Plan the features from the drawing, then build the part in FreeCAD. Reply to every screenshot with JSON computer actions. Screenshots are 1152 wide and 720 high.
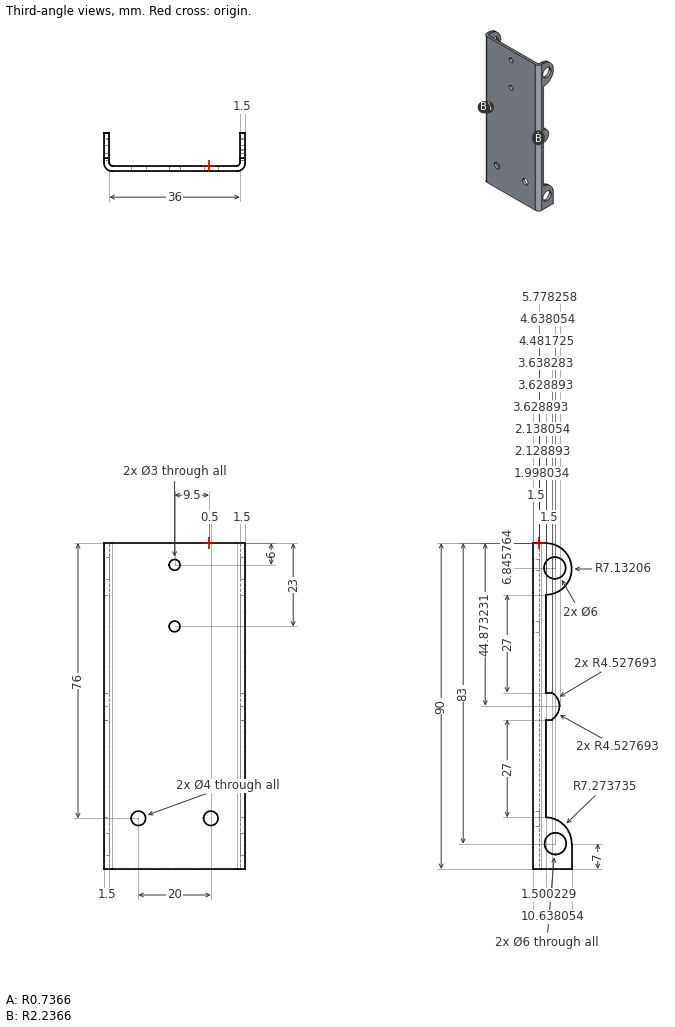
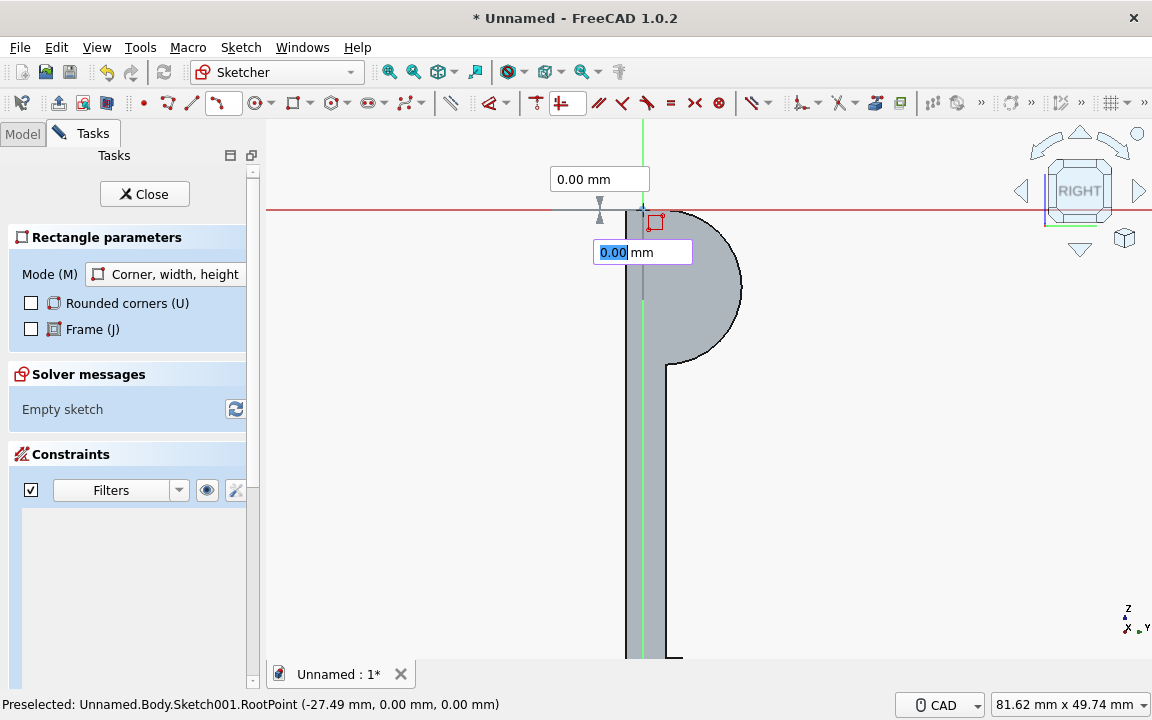
{"action": "scroll", "coordinate": [644, 209], "scroll_direction": "down", "scroll_amount": 5}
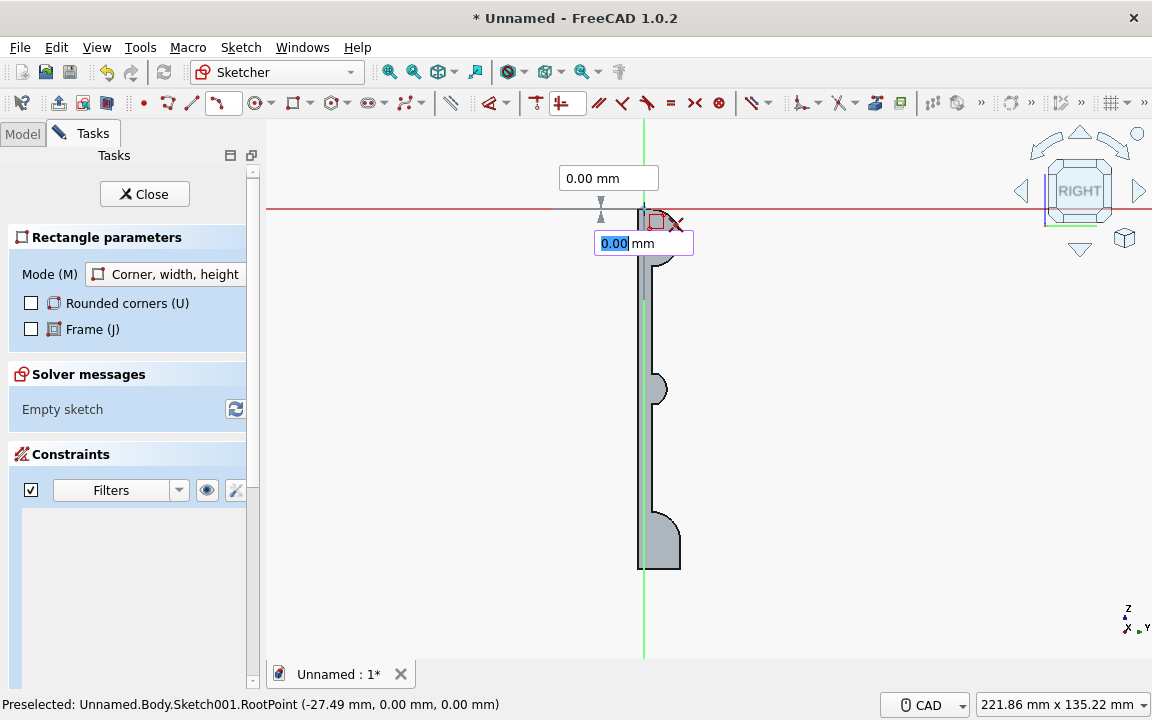
{"action": "scroll", "coordinate": [638, 569], "scroll_direction": "up", "scroll_amount": 5}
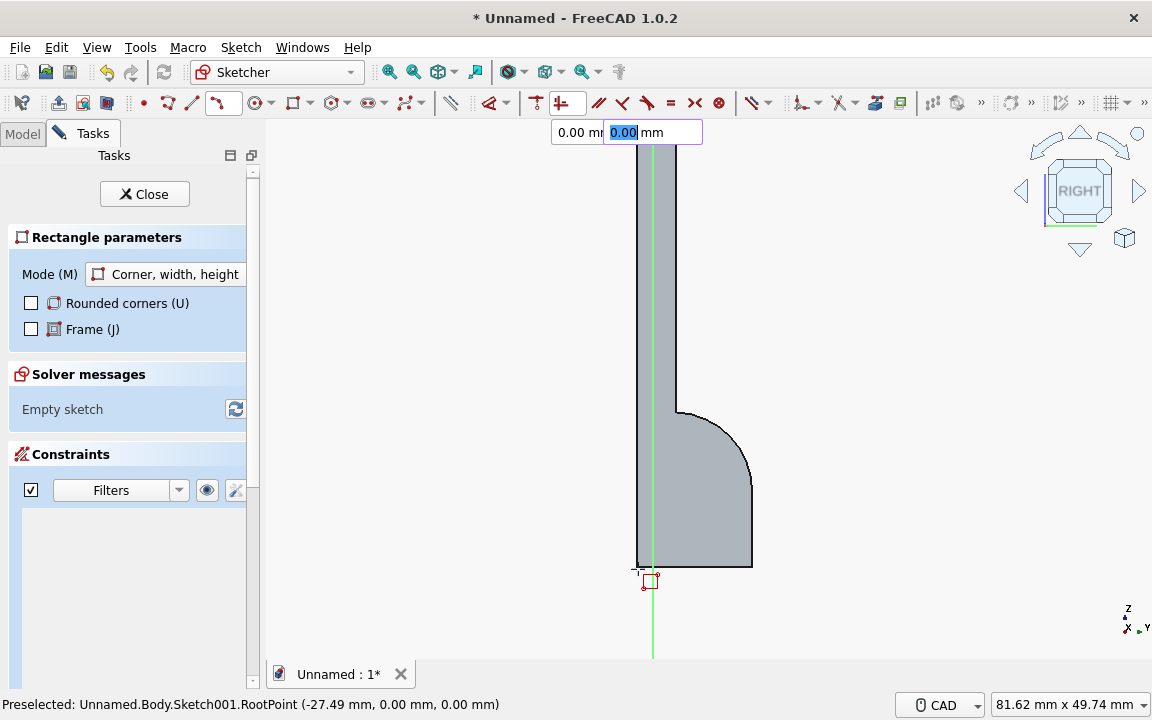
{"action": "left_click", "coordinate": [637, 567]}
{"action": "key", "text": "Escape"}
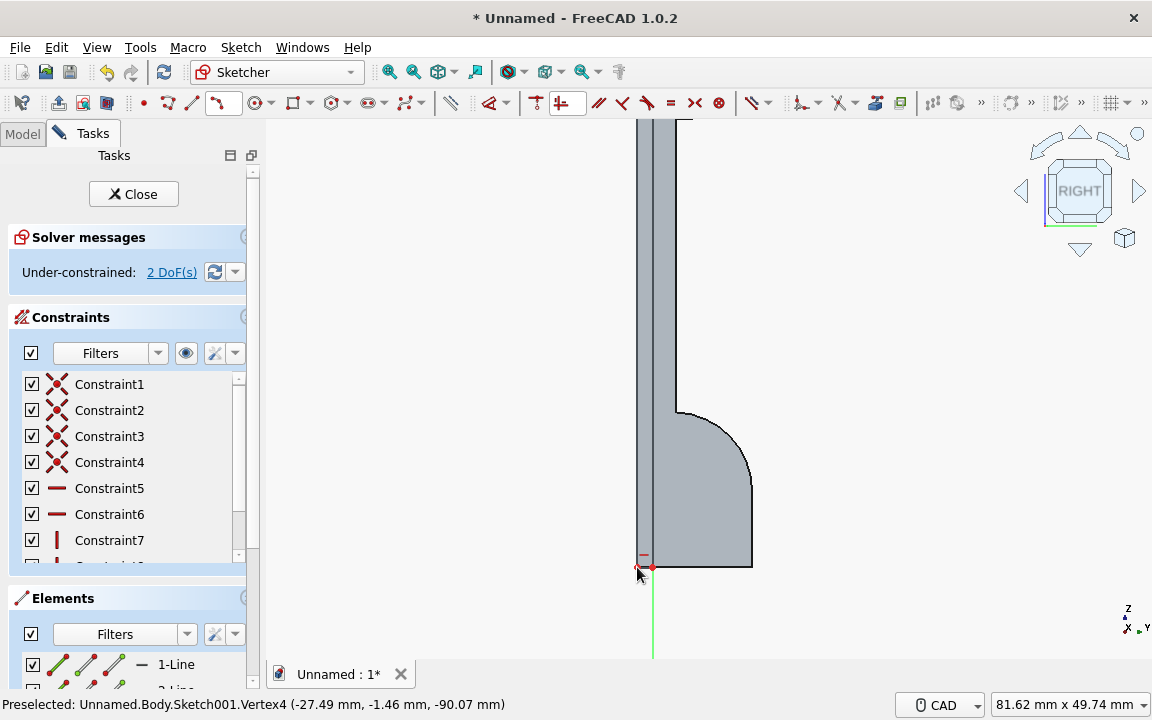
{"action": "key", "text": "d"}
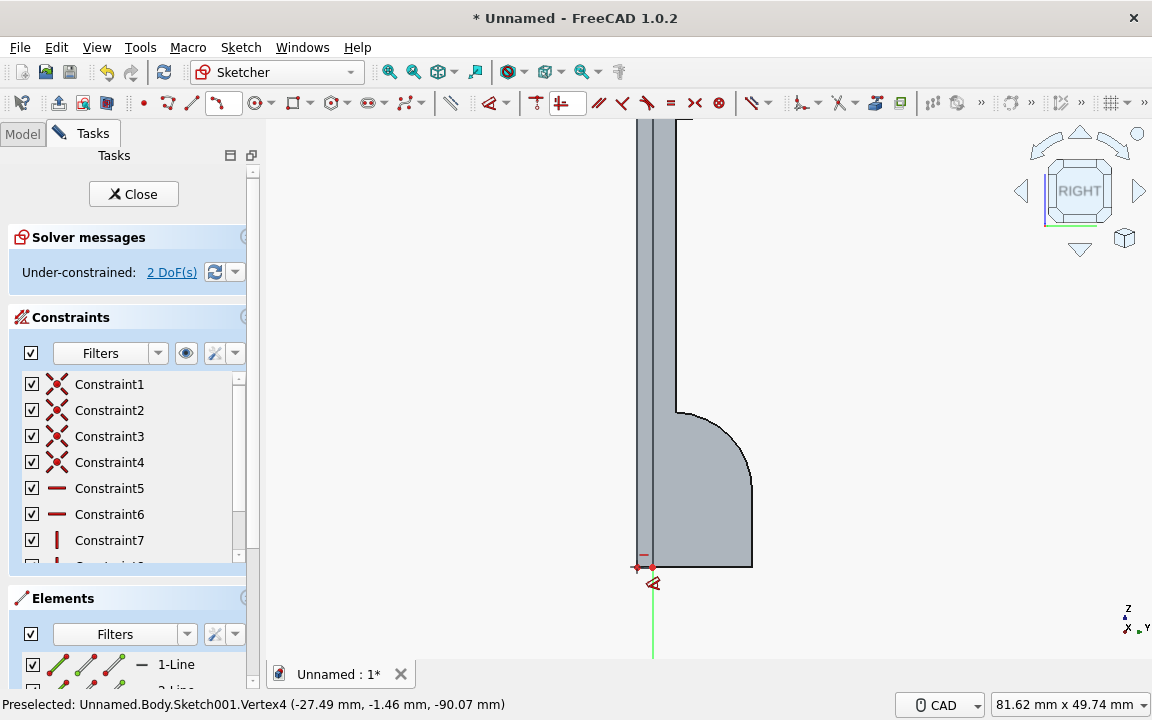
{"action": "left_click", "coordinate": [637, 275]}
{"action": "left_click", "coordinate": [603, 357]}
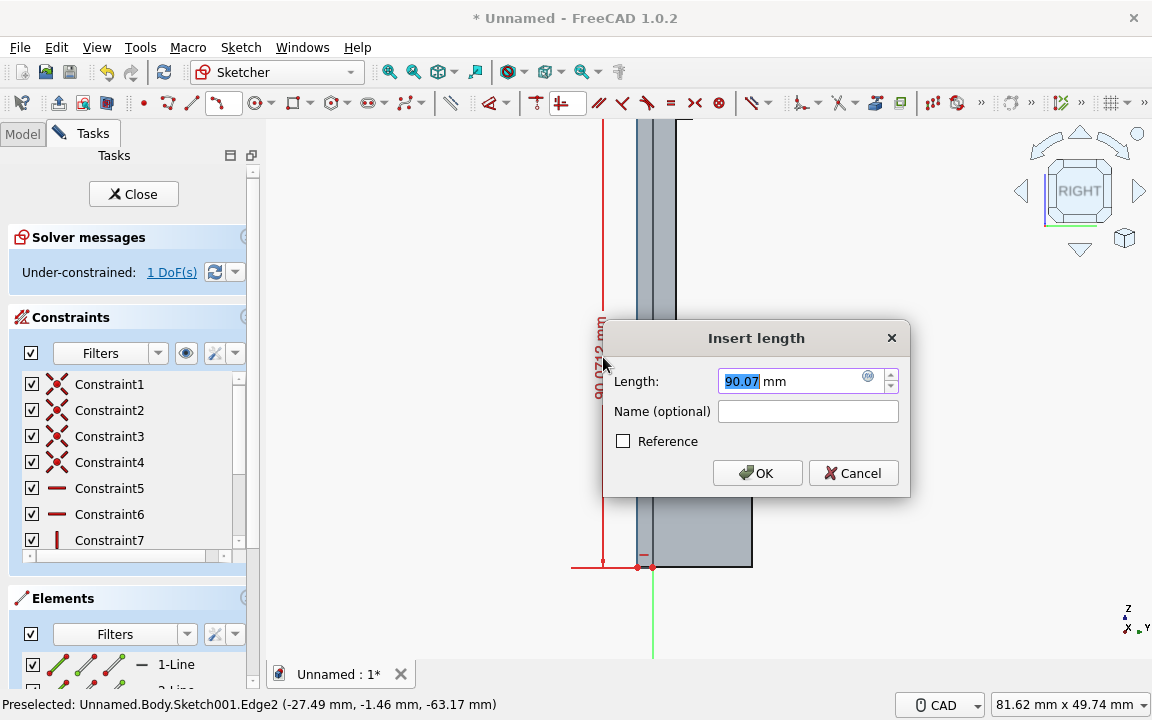
{"action": "type", "text": "90"}
{"action": "key", "text": "Return"}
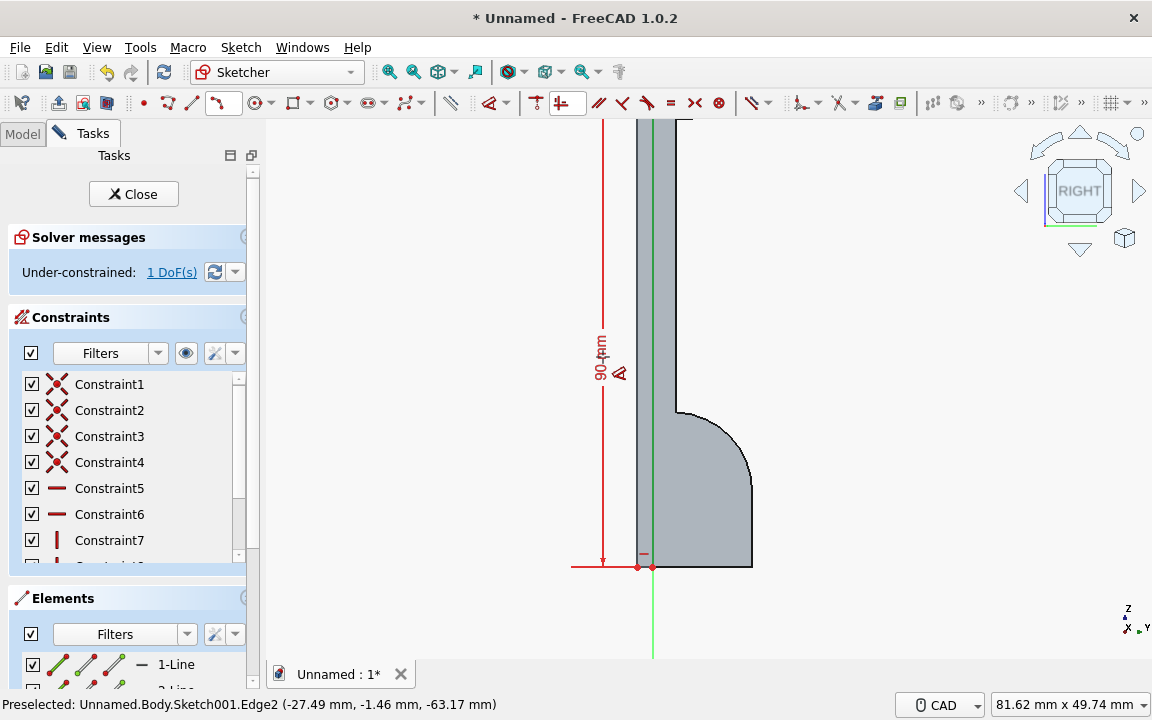
{"action": "scroll", "coordinate": [638, 570], "scroll_direction": "down", "scroll_amount": 5}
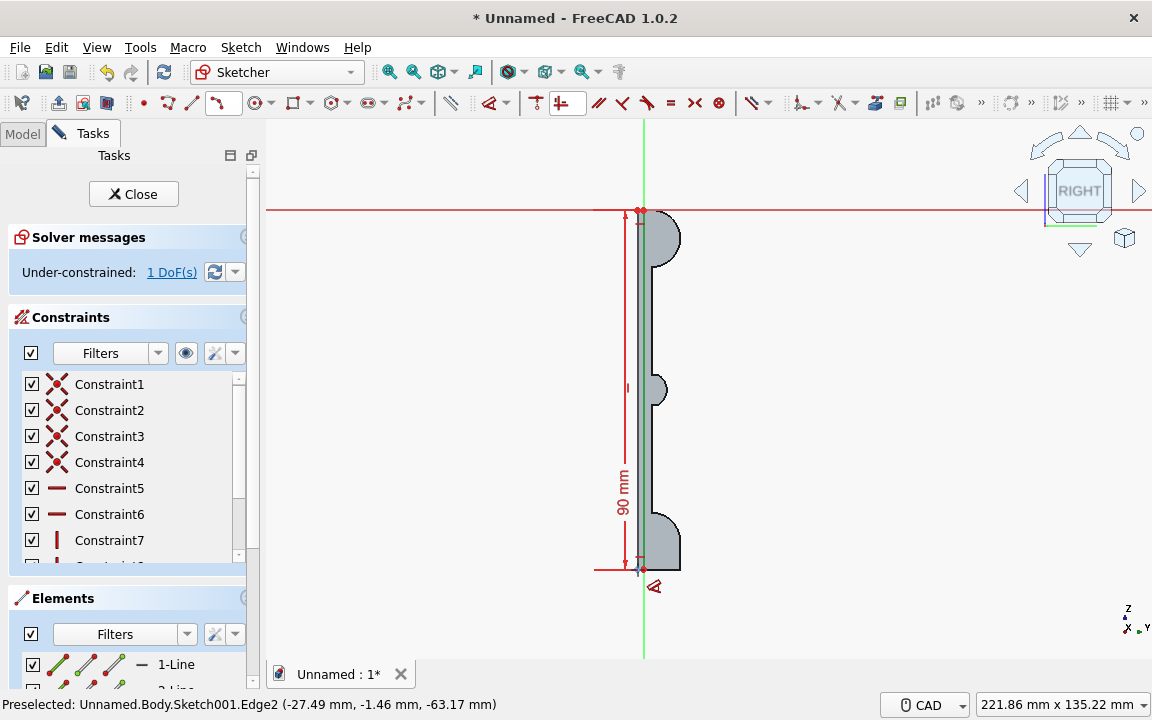
{"action": "scroll", "coordinate": [641, 210], "scroll_direction": "up", "scroll_amount": 10}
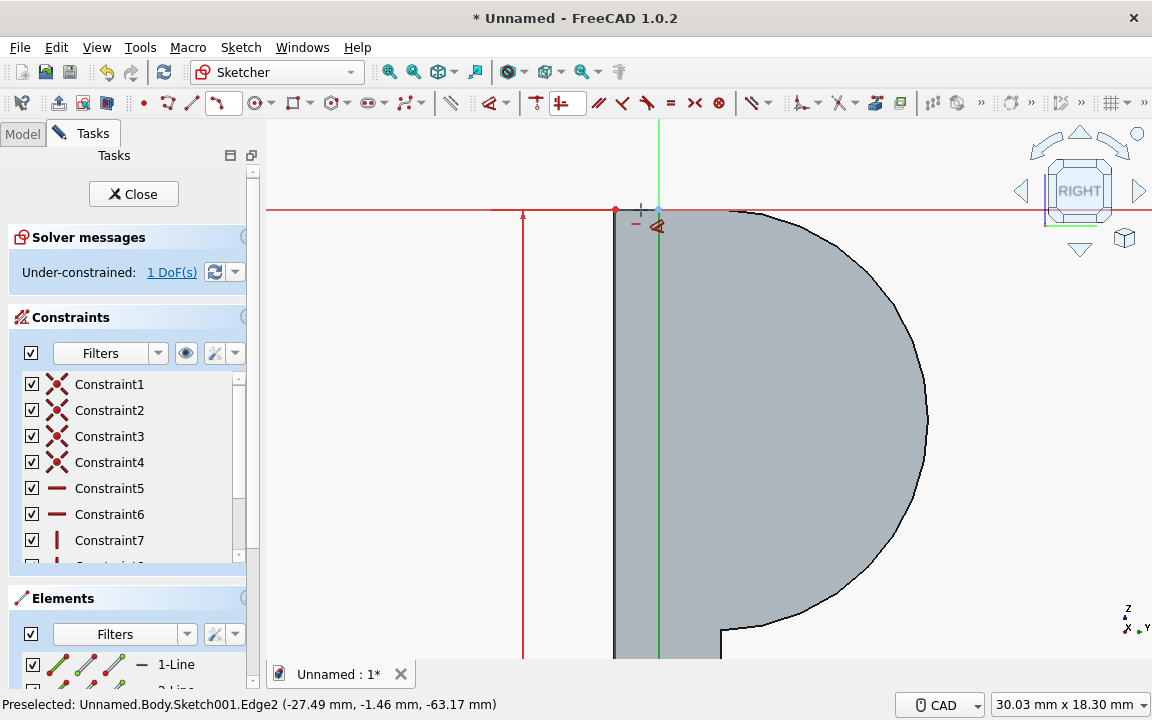
{"action": "left_click", "coordinate": [637, 210]}
{"action": "left_click", "coordinate": [637, 176]}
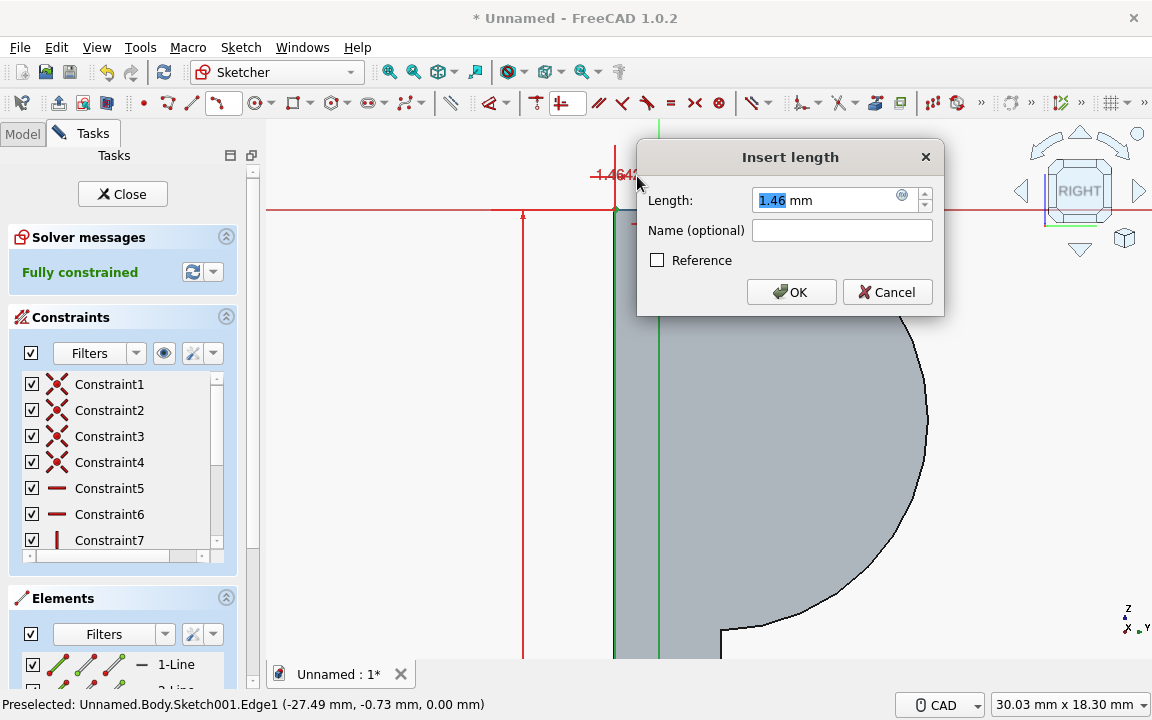
{"action": "type", "text": "1.5"}
{"action": "key", "text": "Return"}
{"action": "key", "text": "Escape"}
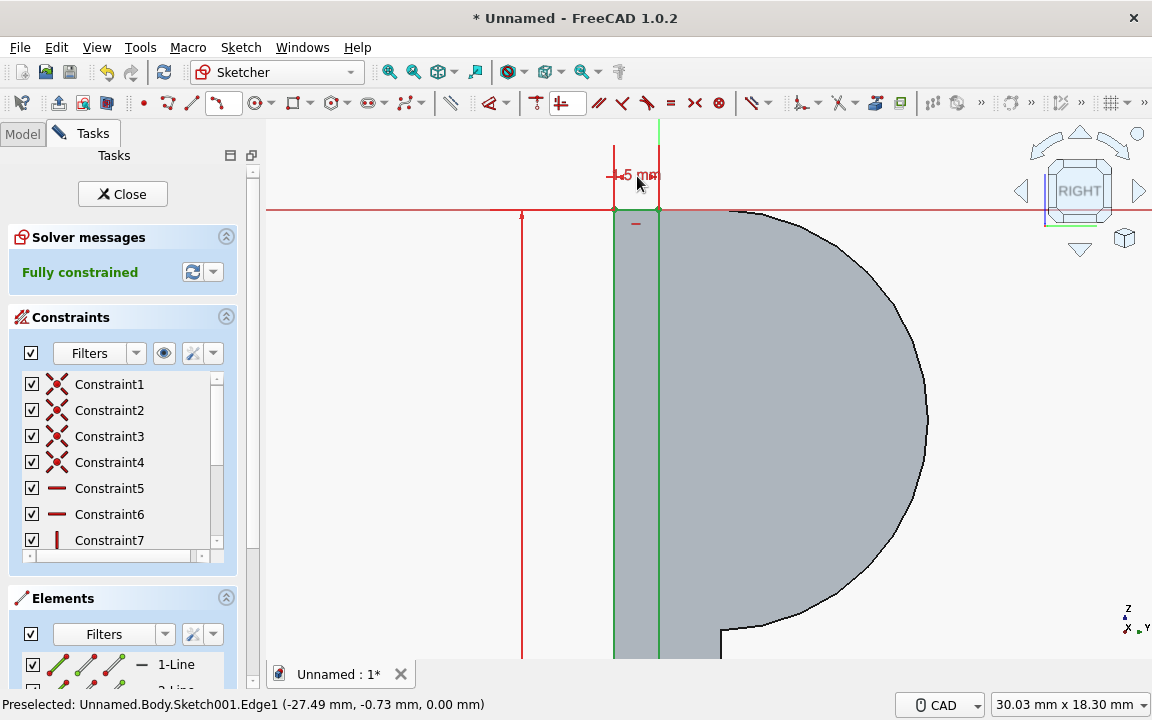
{"action": "left_click", "coordinate": [123, 194]}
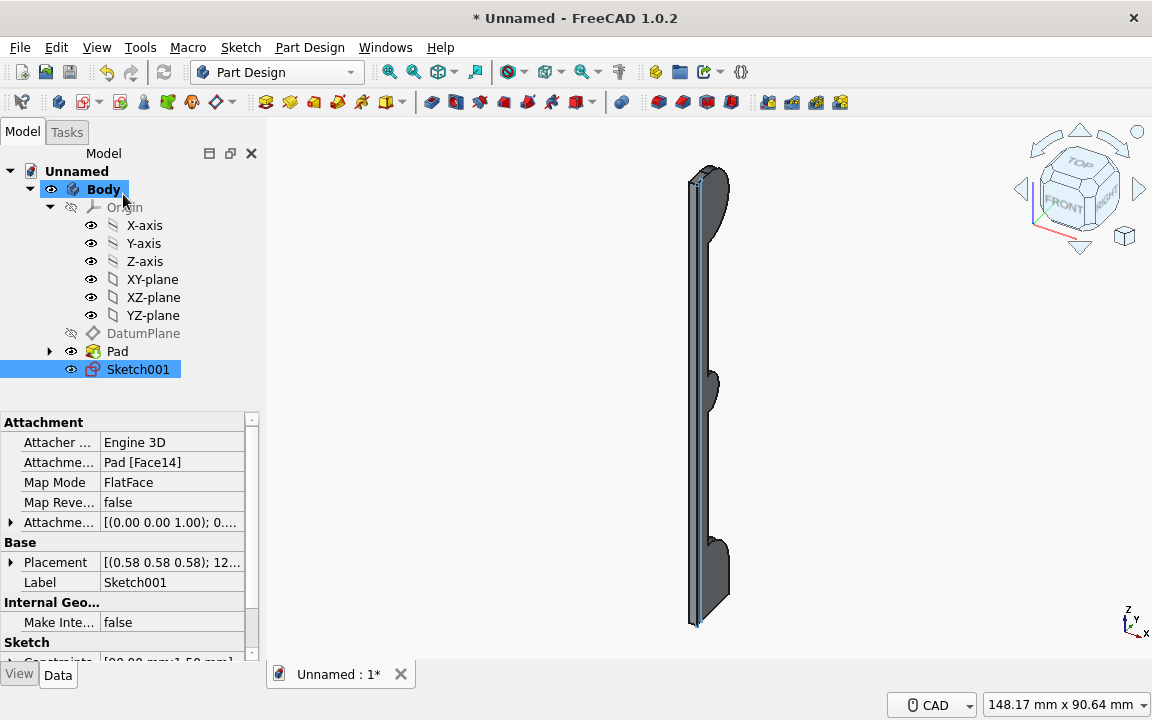
{"action": "left_click", "coordinate": [266, 102]}